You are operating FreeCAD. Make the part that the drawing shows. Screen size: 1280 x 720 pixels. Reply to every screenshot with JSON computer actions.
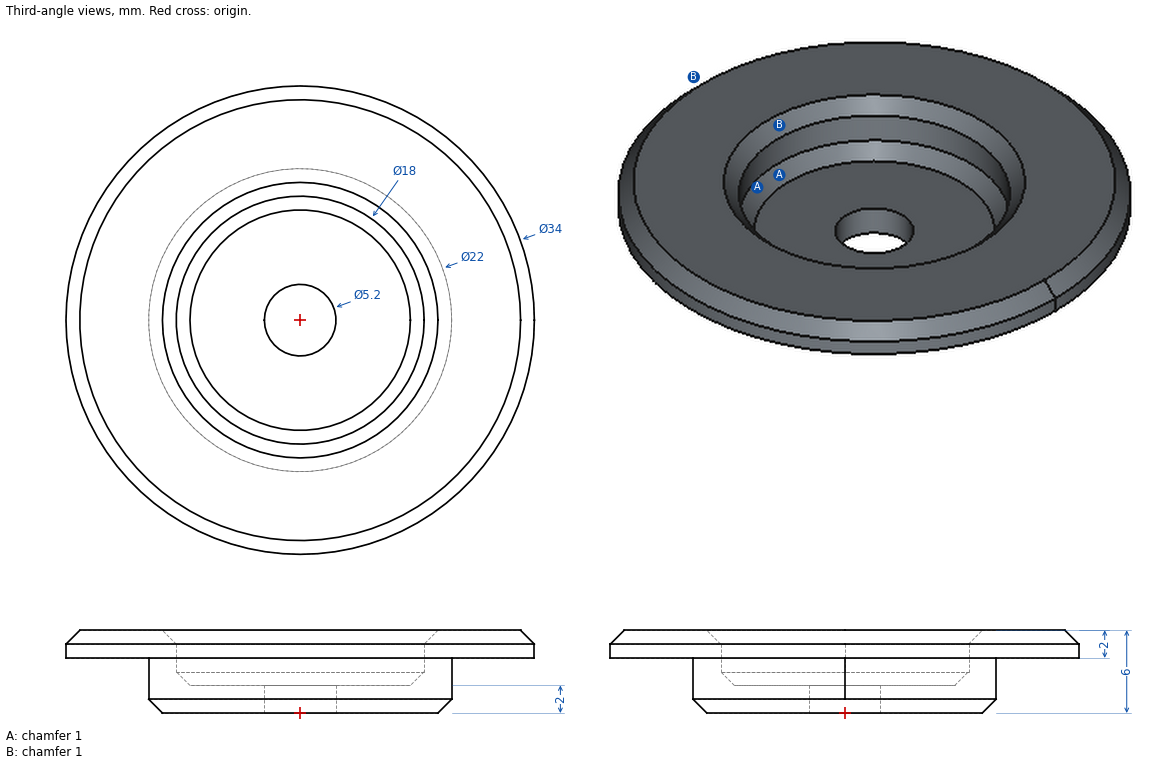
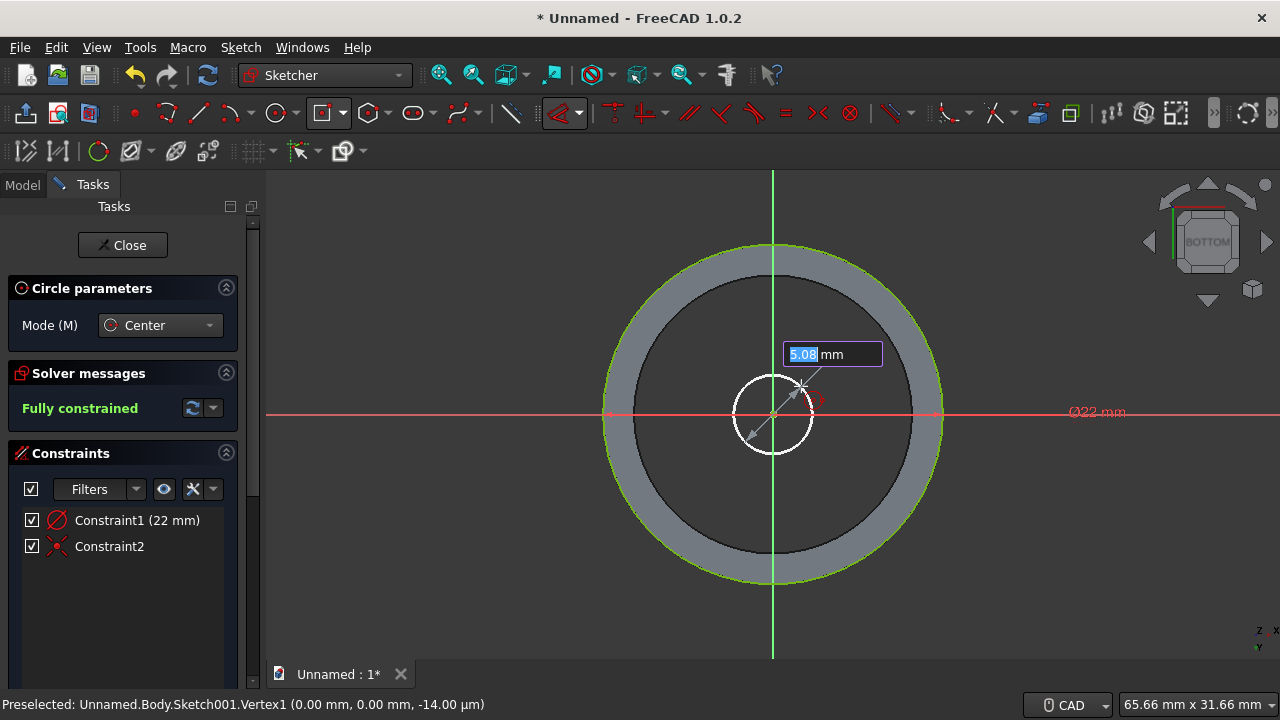
{"action": "type", "text": "5.2"}
{"action": "key", "text": "Return"}
{"action": "key", "text": "Escape"}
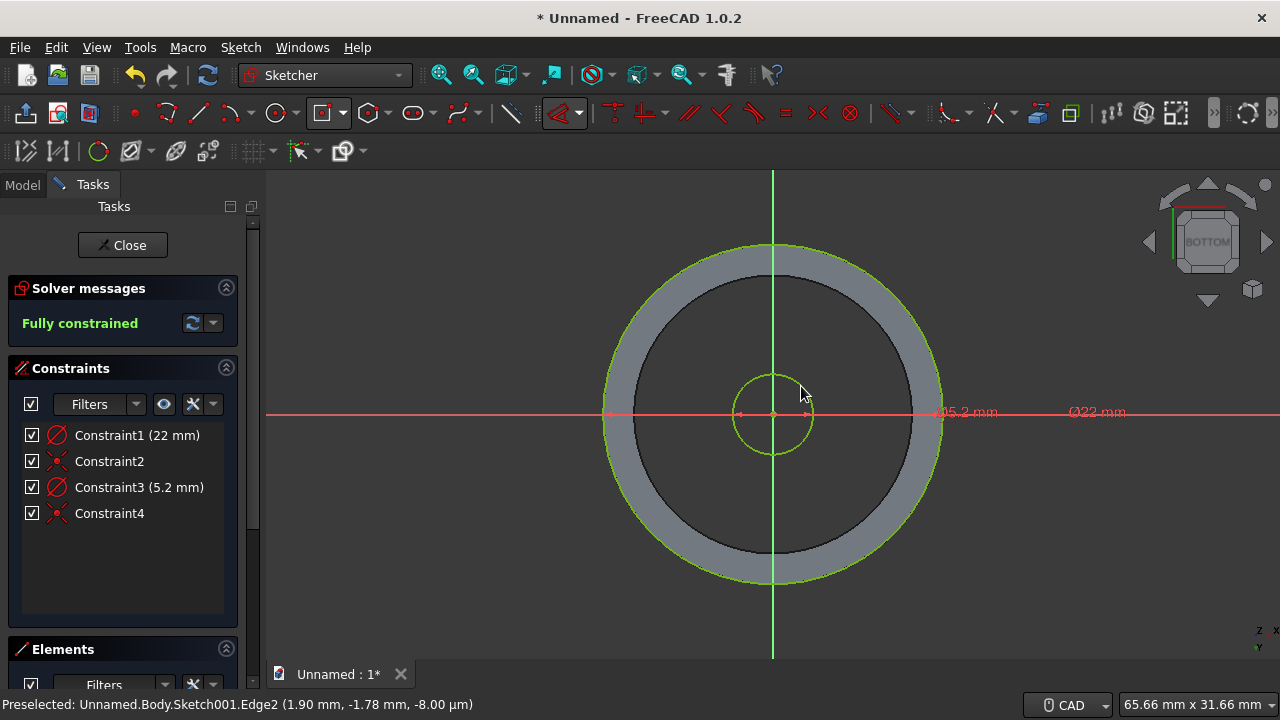
{"action": "left_click", "coordinate": [123, 245]}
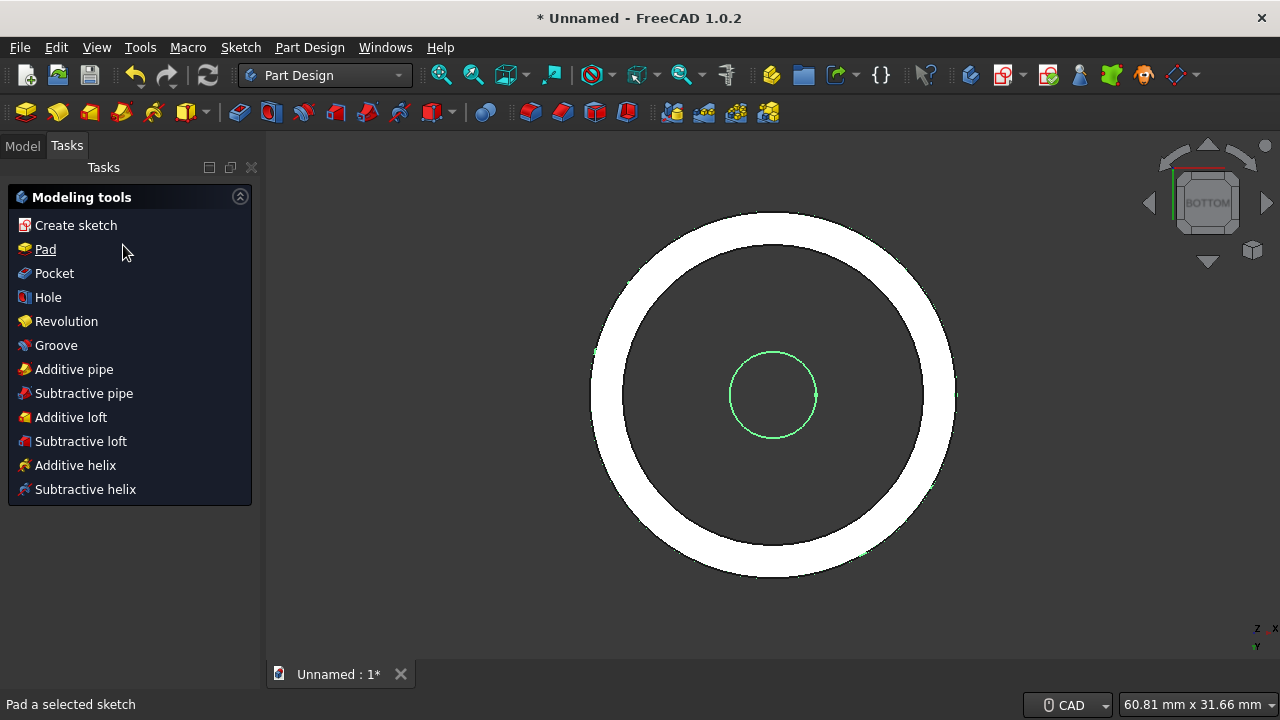
{"action": "left_click", "coordinate": [26, 112]}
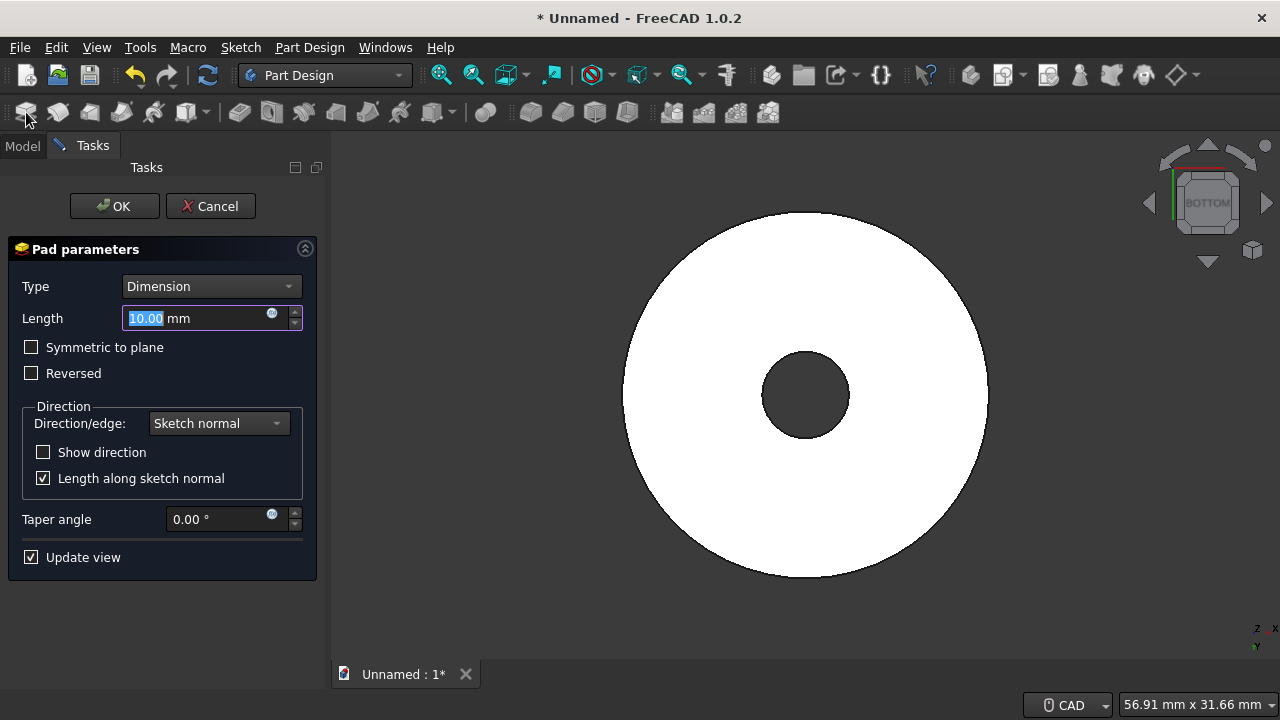
{"action": "type", "text": "2"}
{"action": "key", "text": "Tab"}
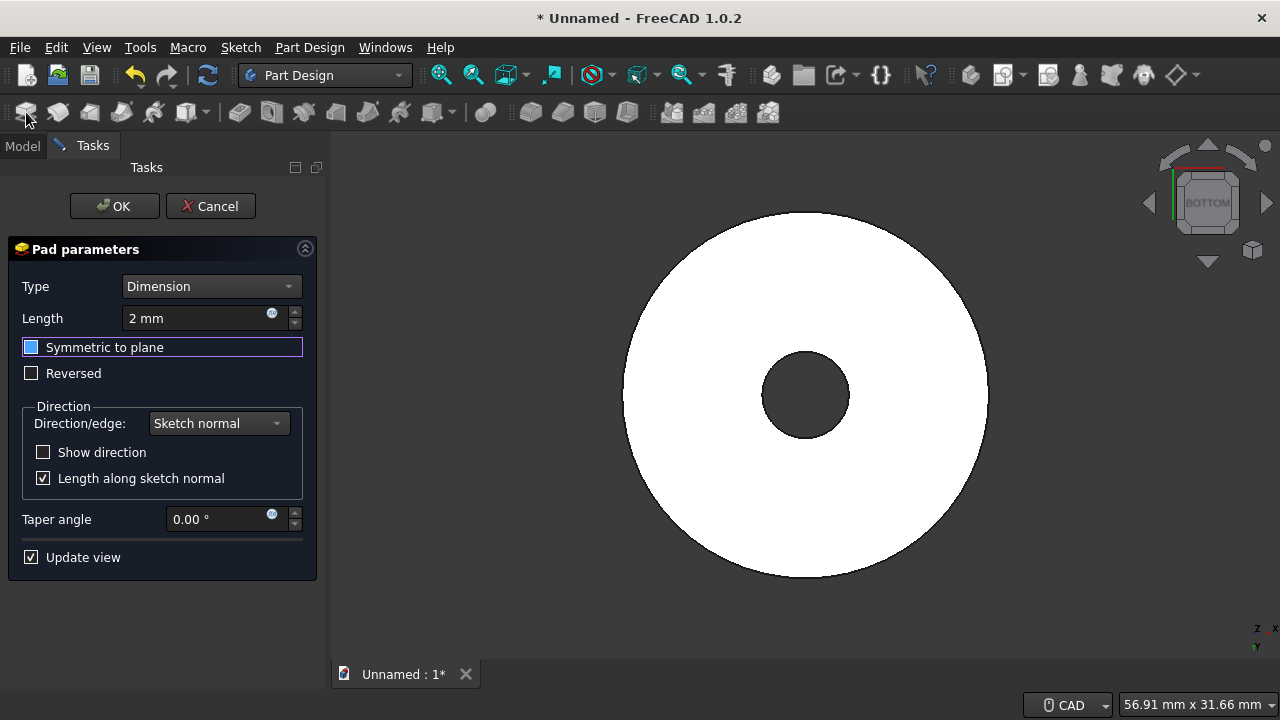
{"action": "left_click", "coordinate": [30, 373]}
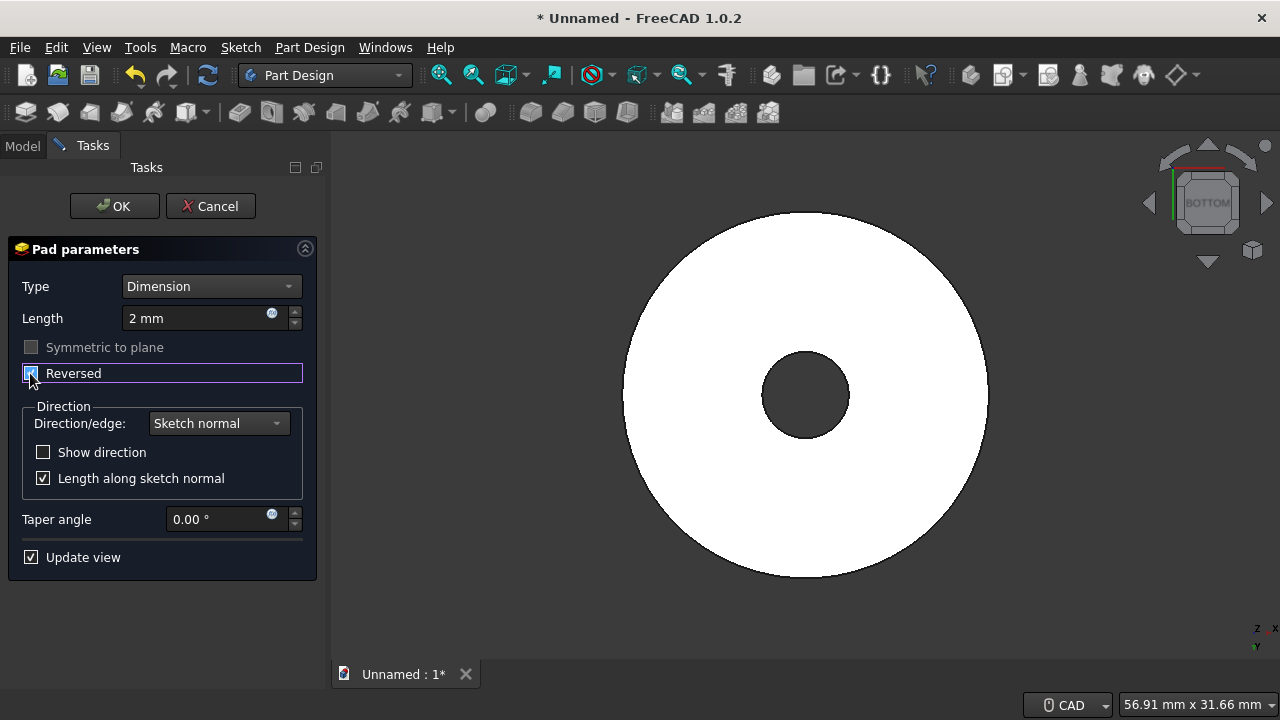
{"action": "left_click", "coordinate": [115, 206]}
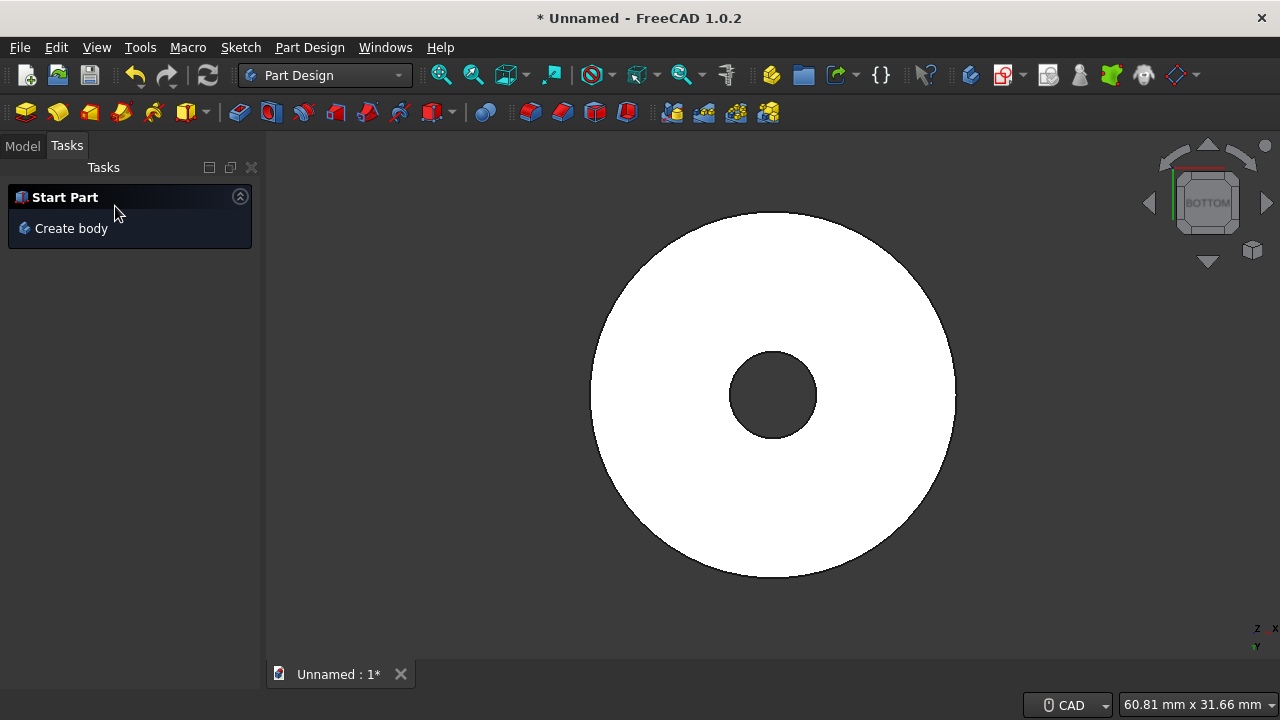
{"action": "left_click", "coordinate": [590, 394]}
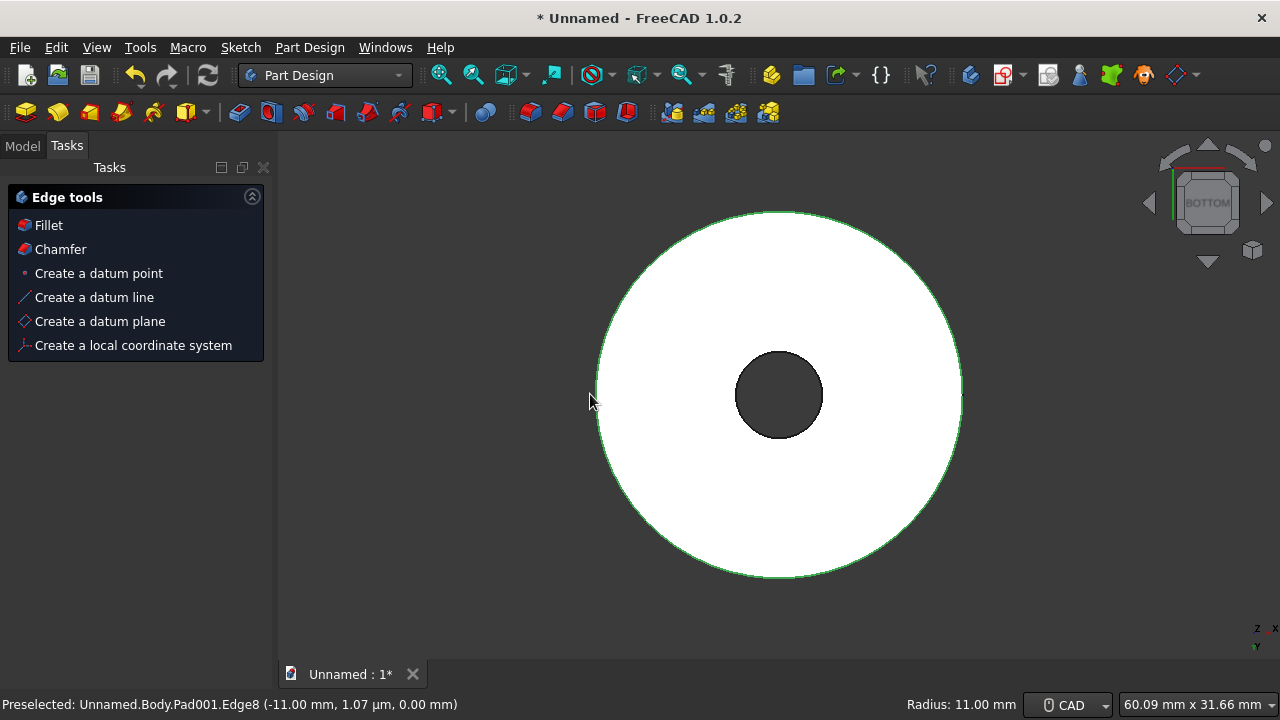
{"action": "key", "text": "0"}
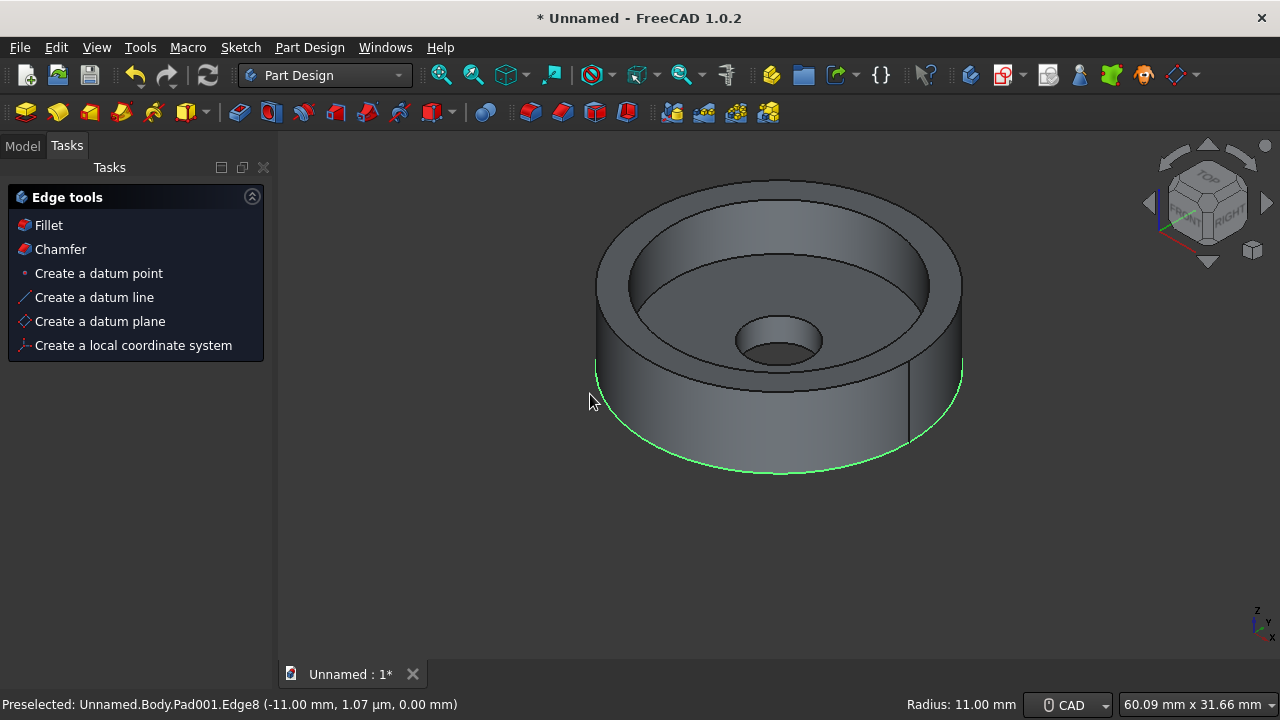
{"action": "key", "text": "2"}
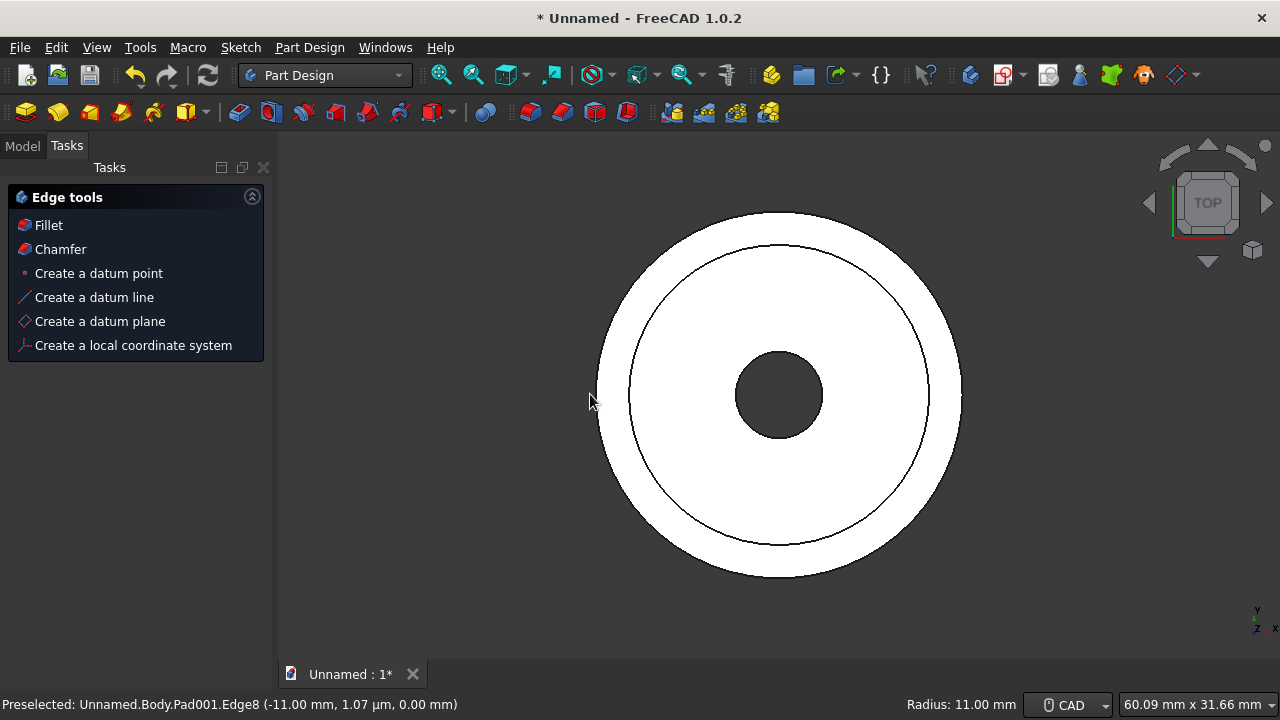
{"action": "key", "text": "1"}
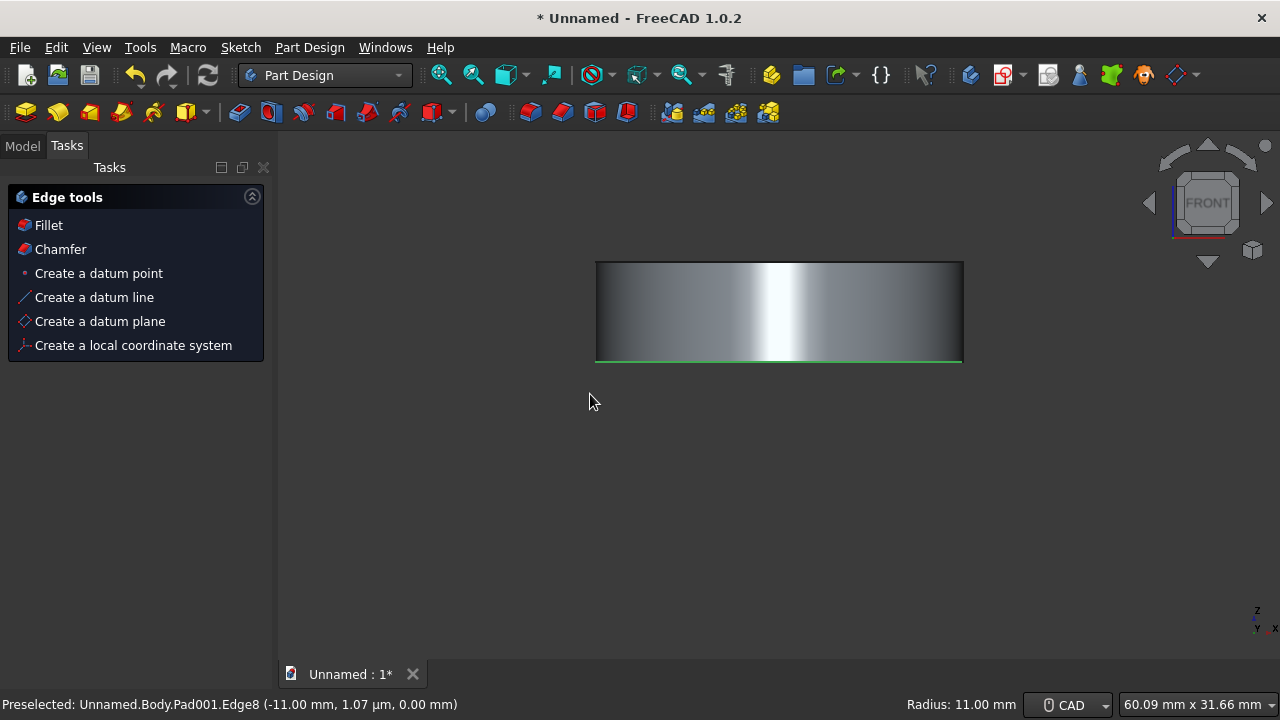
{"action": "left_click", "coordinate": [442, 76]}